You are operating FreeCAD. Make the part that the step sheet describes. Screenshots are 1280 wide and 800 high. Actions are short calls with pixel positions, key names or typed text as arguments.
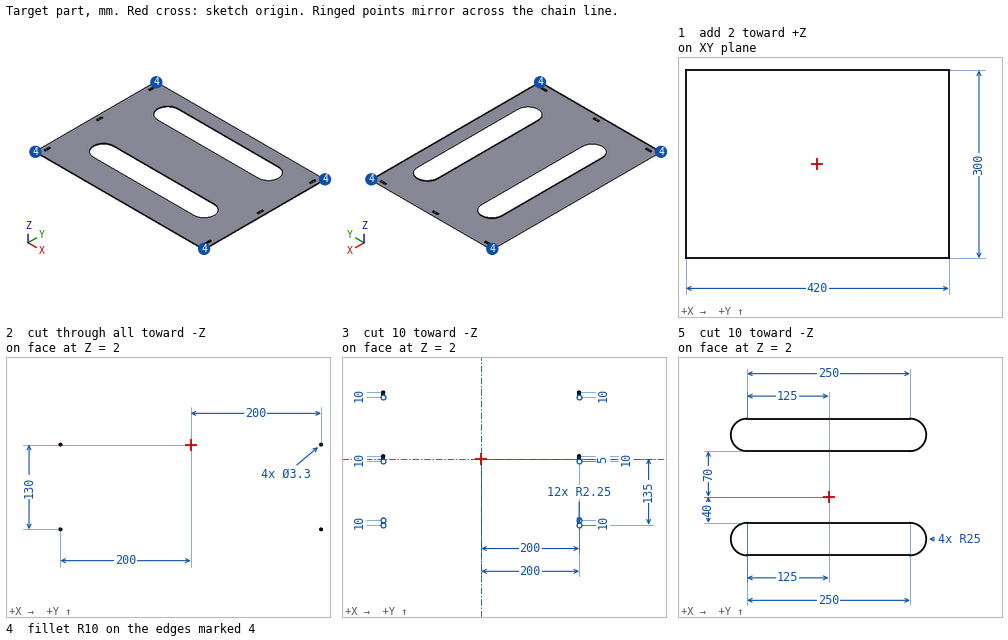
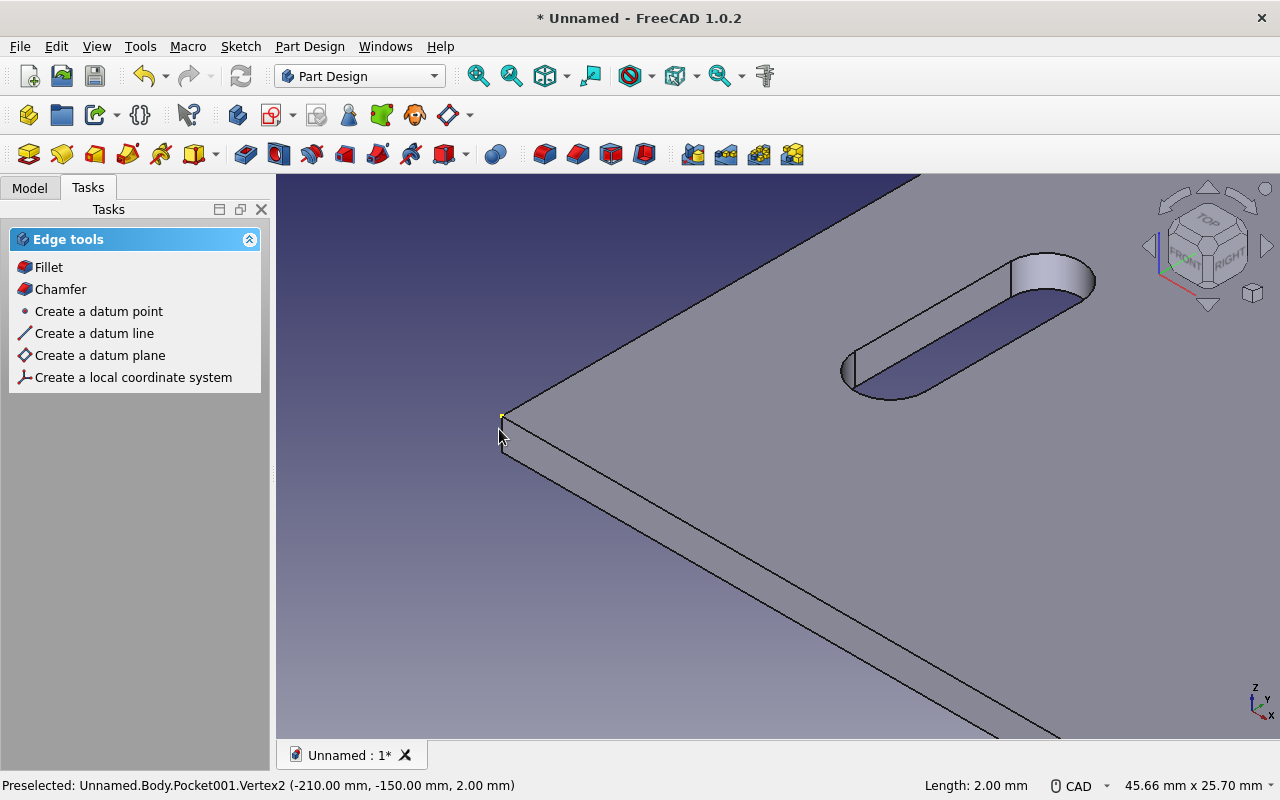
click(479, 76)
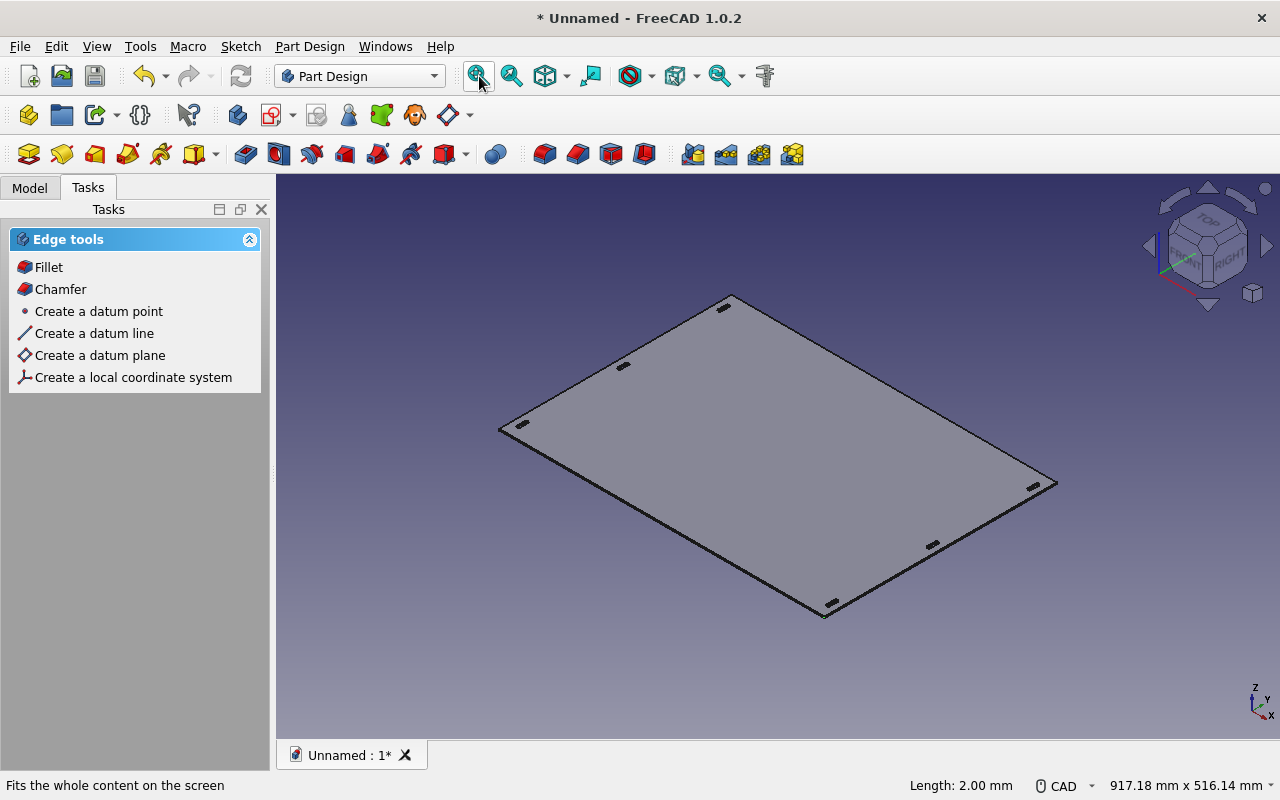
key(2)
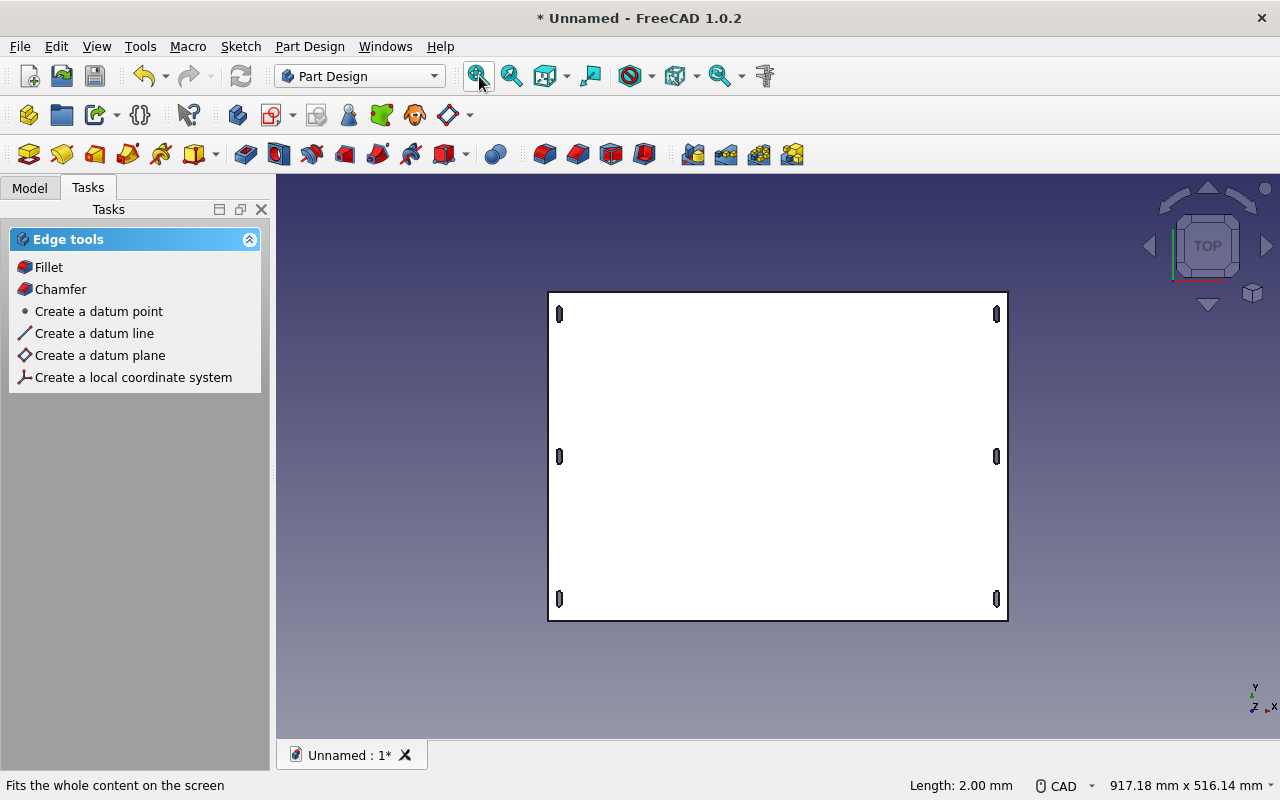
scroll(548, 620, up, 15)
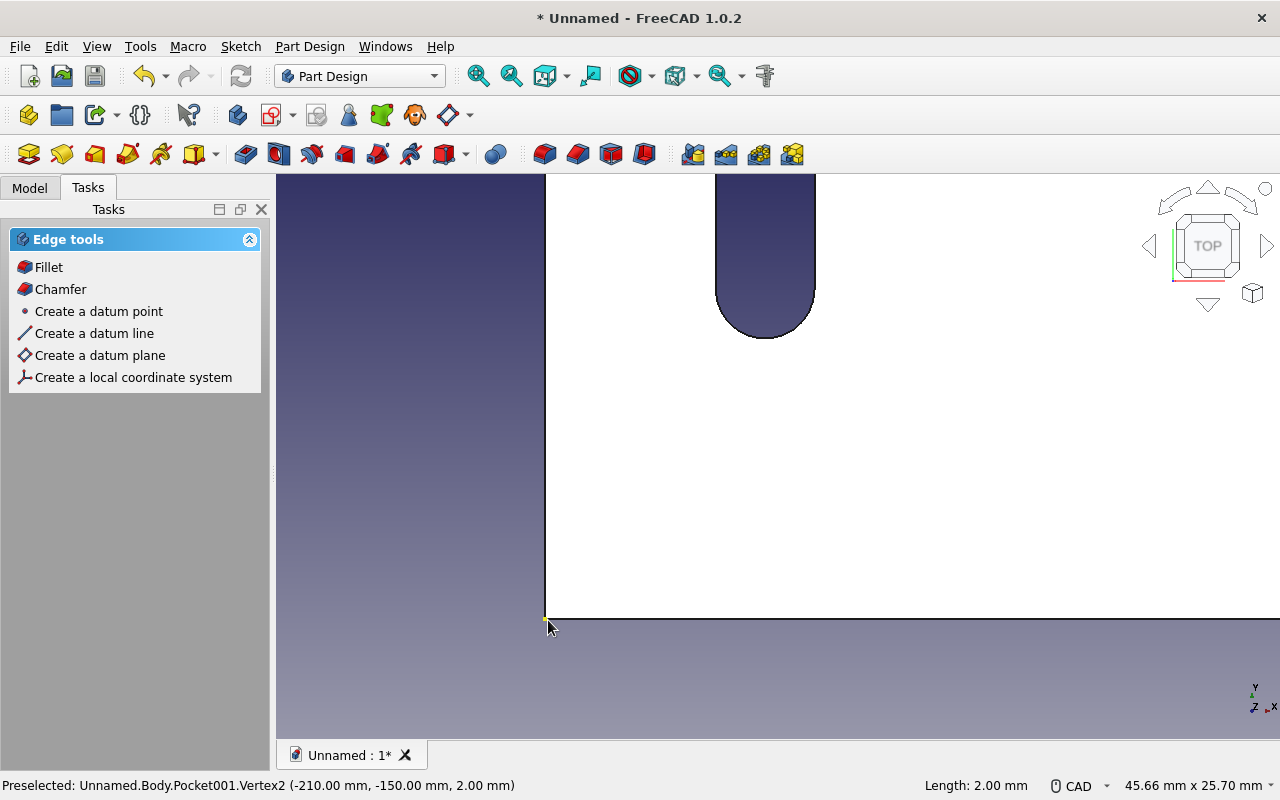
click(479, 76)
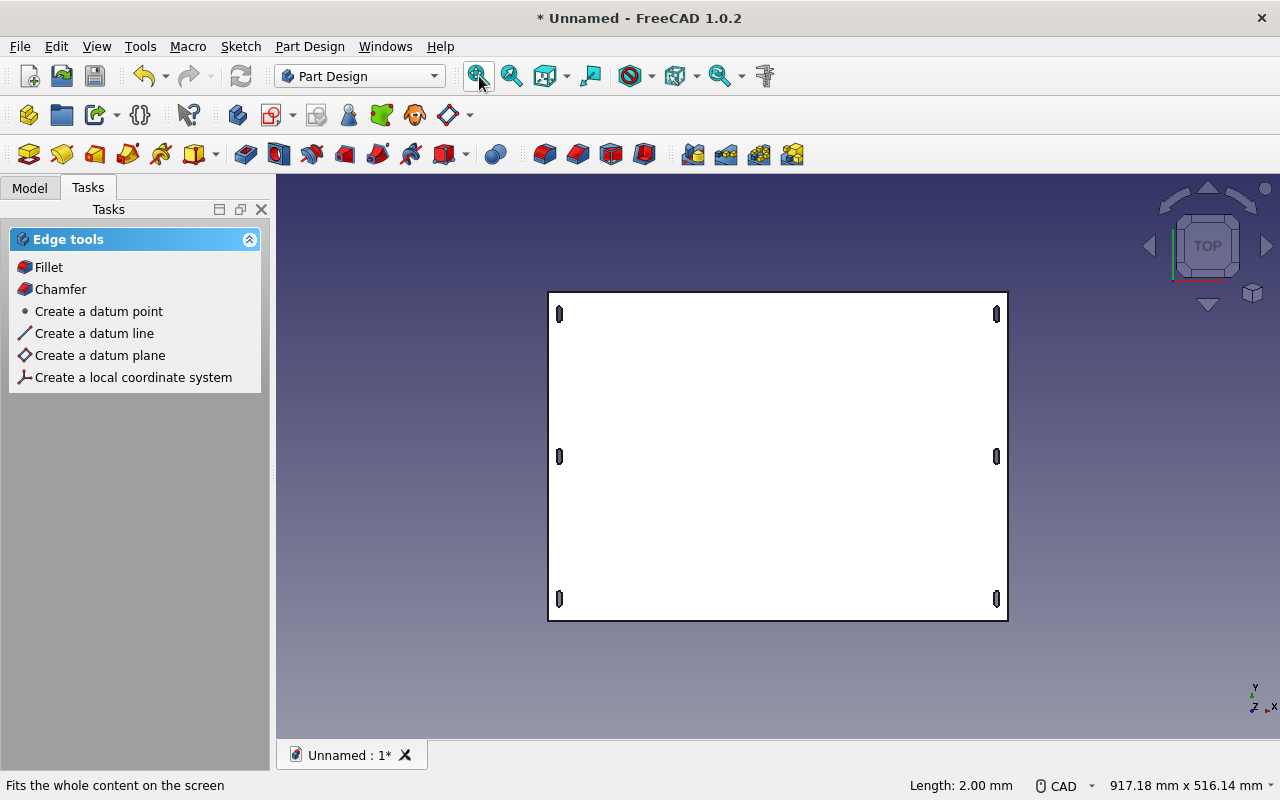
key(1)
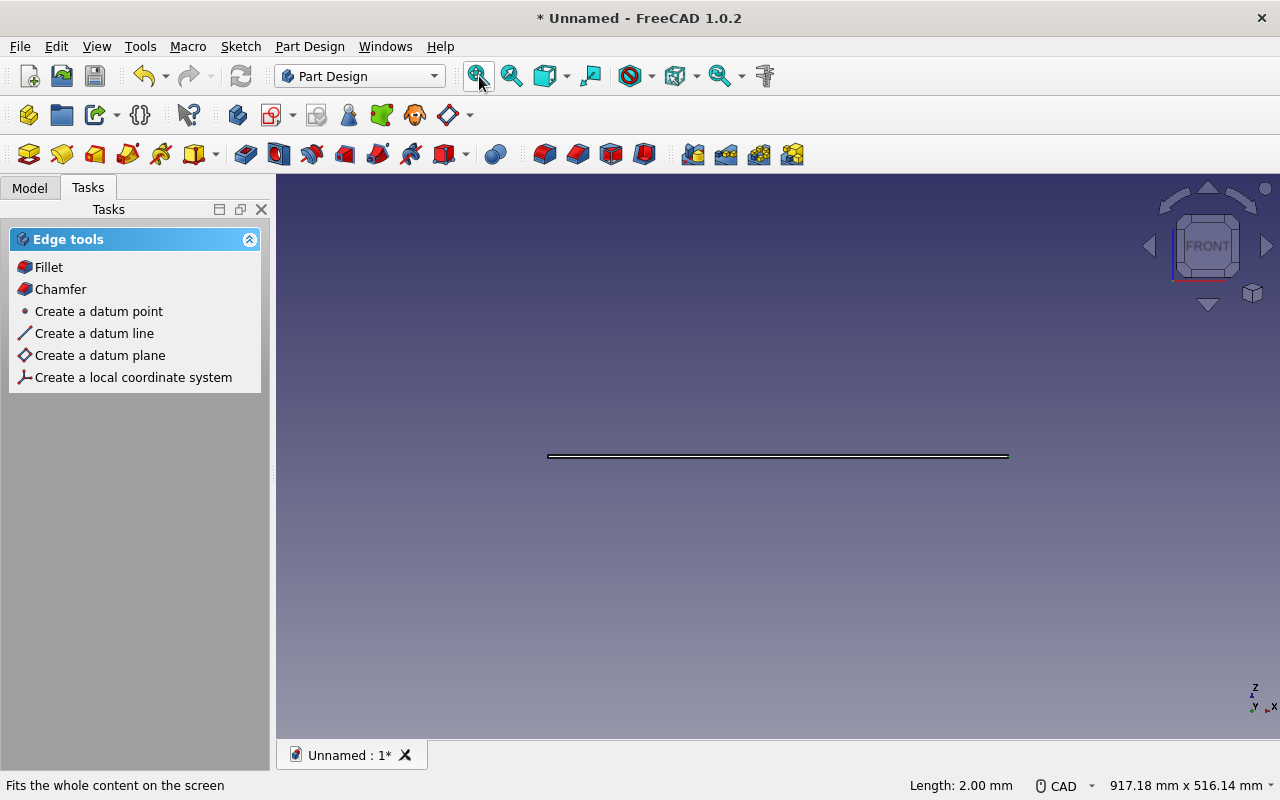
scroll(548, 455, up, 15)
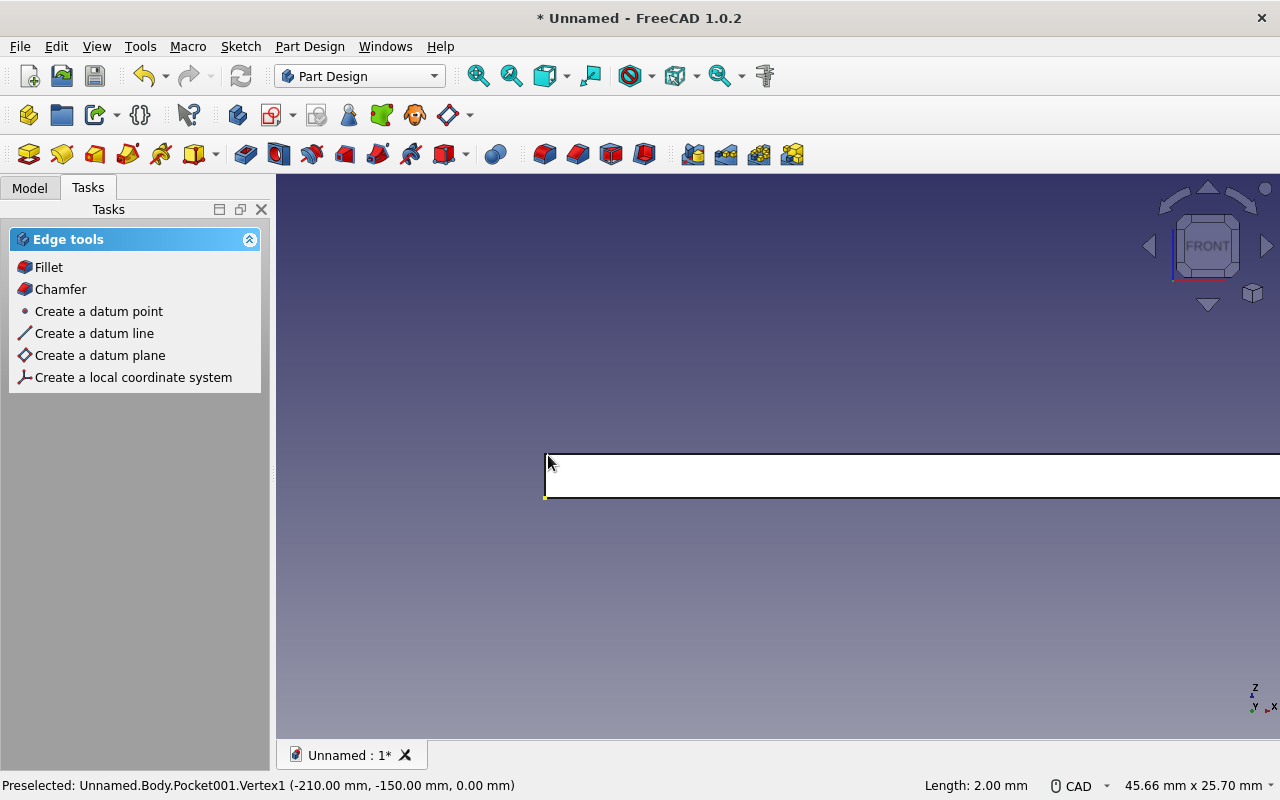
click(545, 475, ctrl)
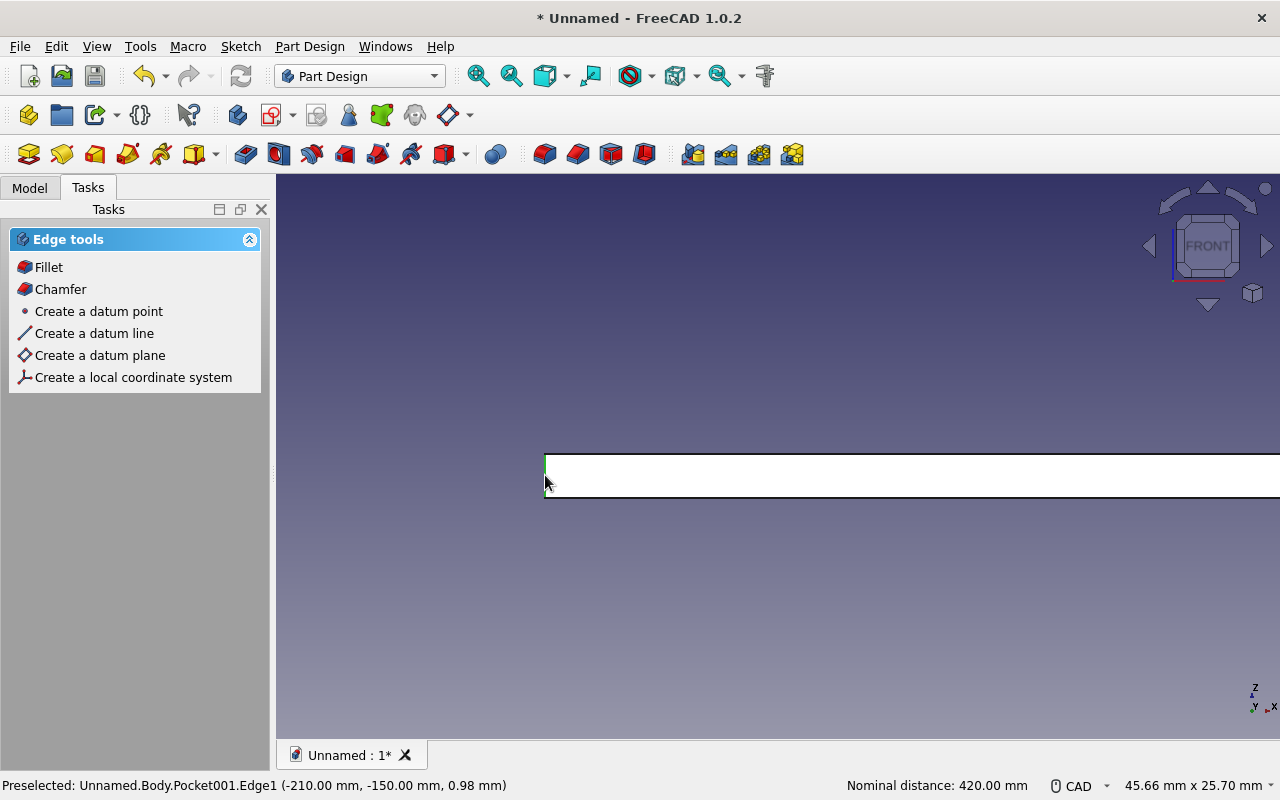
key(v)
key(f)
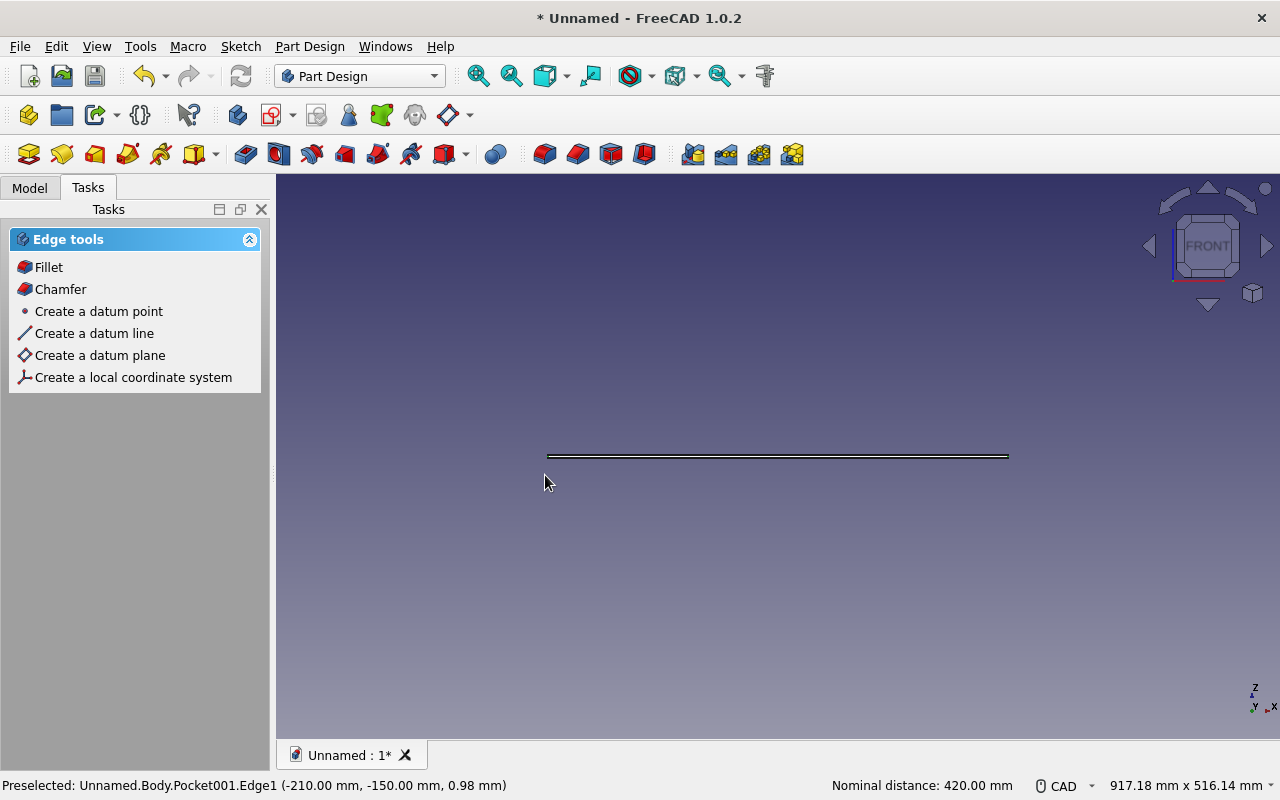
key(3)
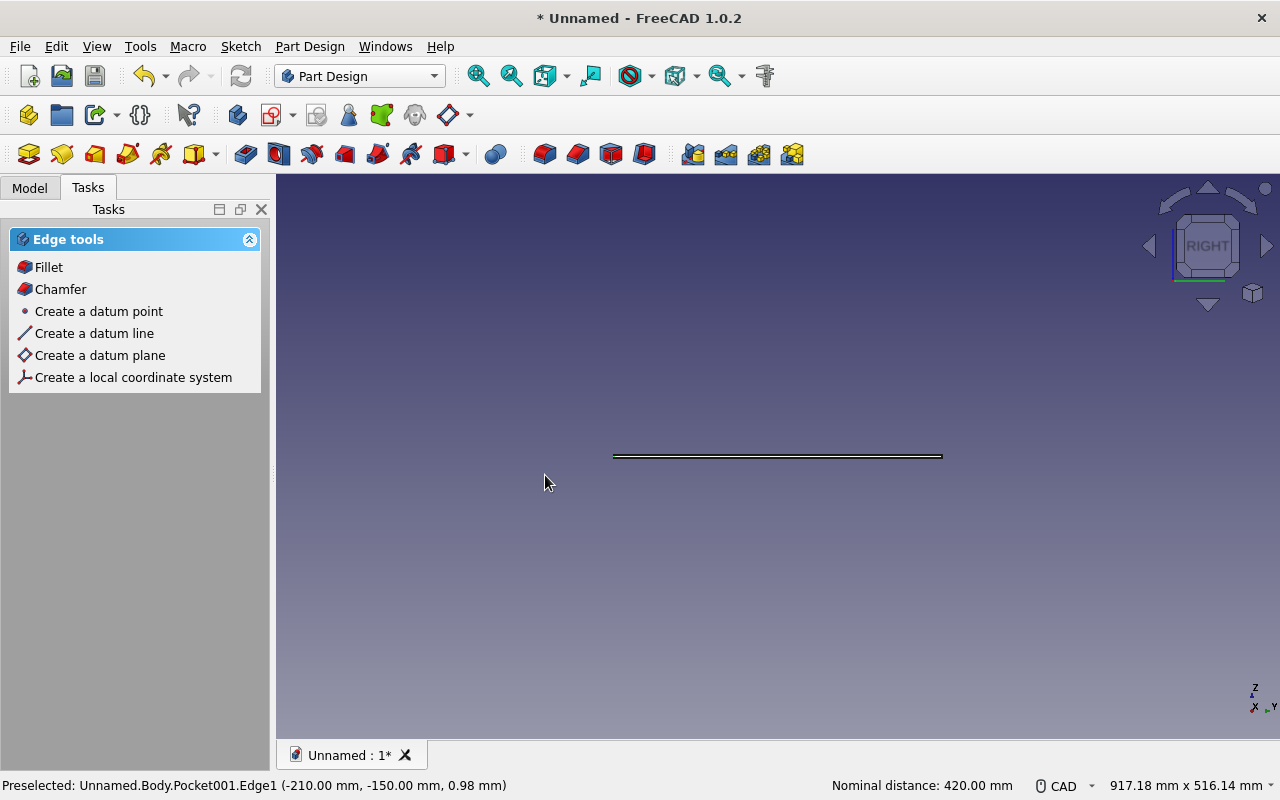
click(479, 76)